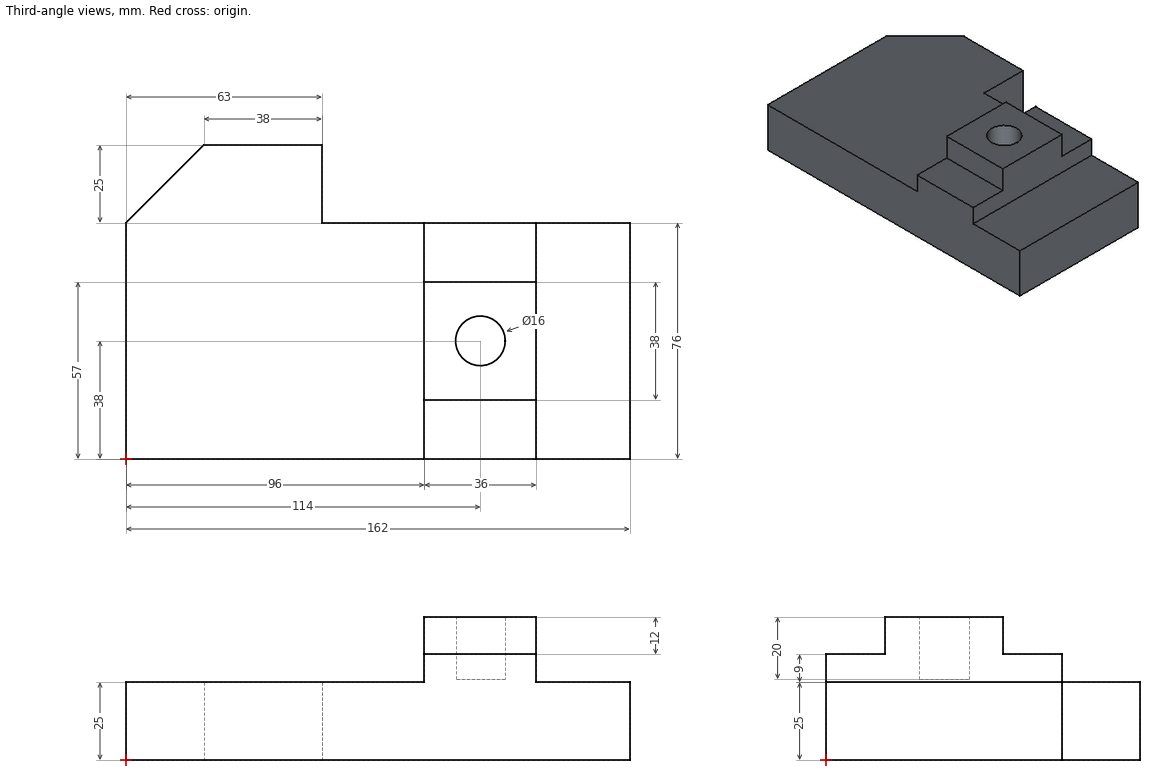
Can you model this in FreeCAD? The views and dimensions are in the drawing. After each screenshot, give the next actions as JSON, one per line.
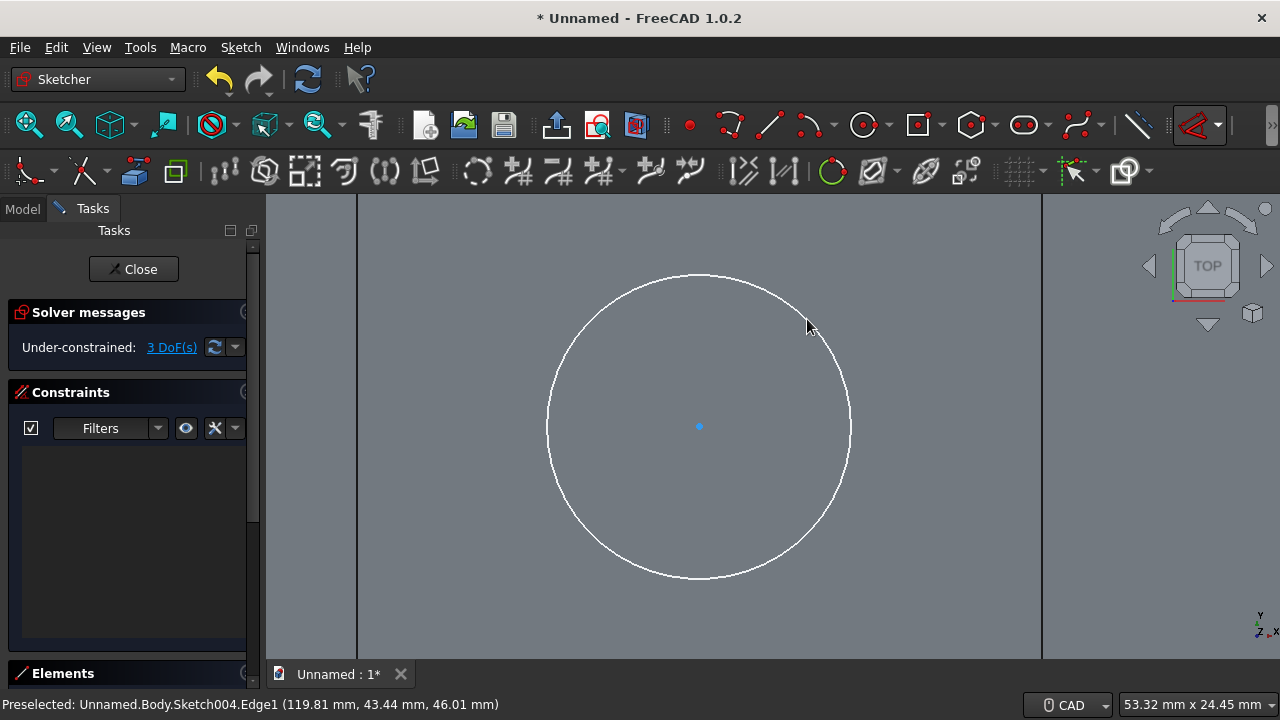
{"action": "left_click", "coordinate": [806, 319]}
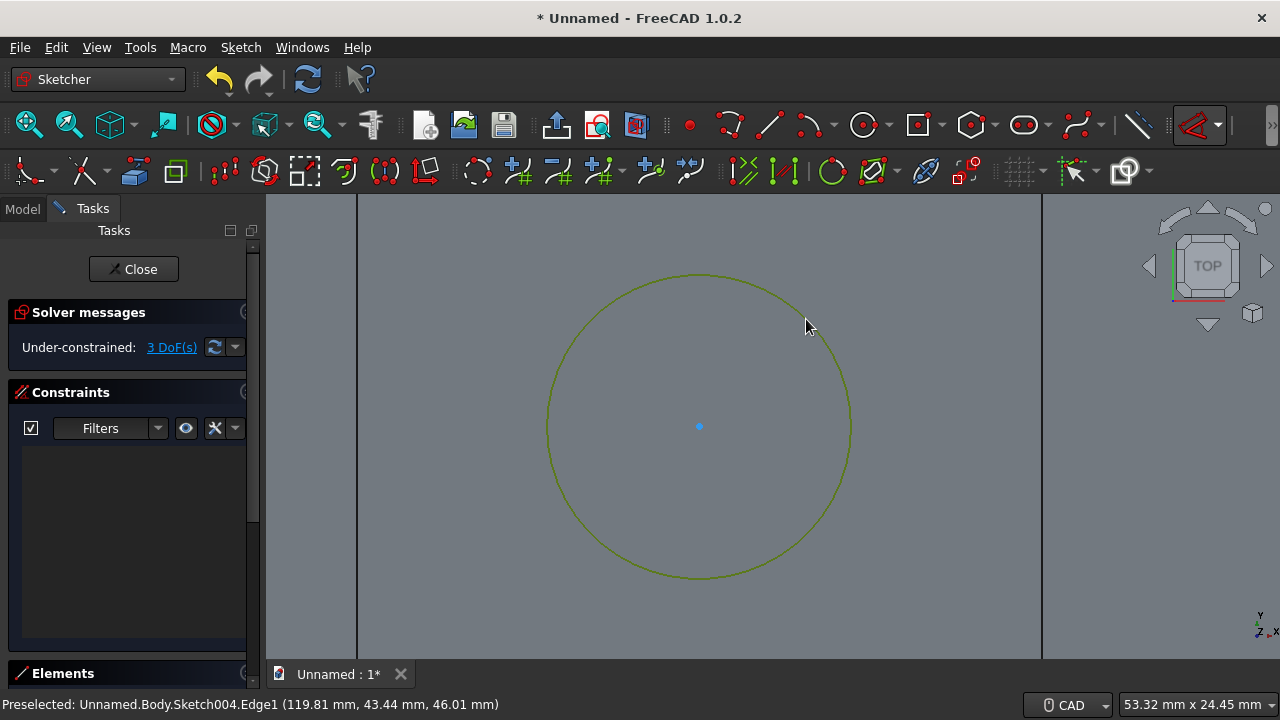
{"action": "key", "text": "k o"}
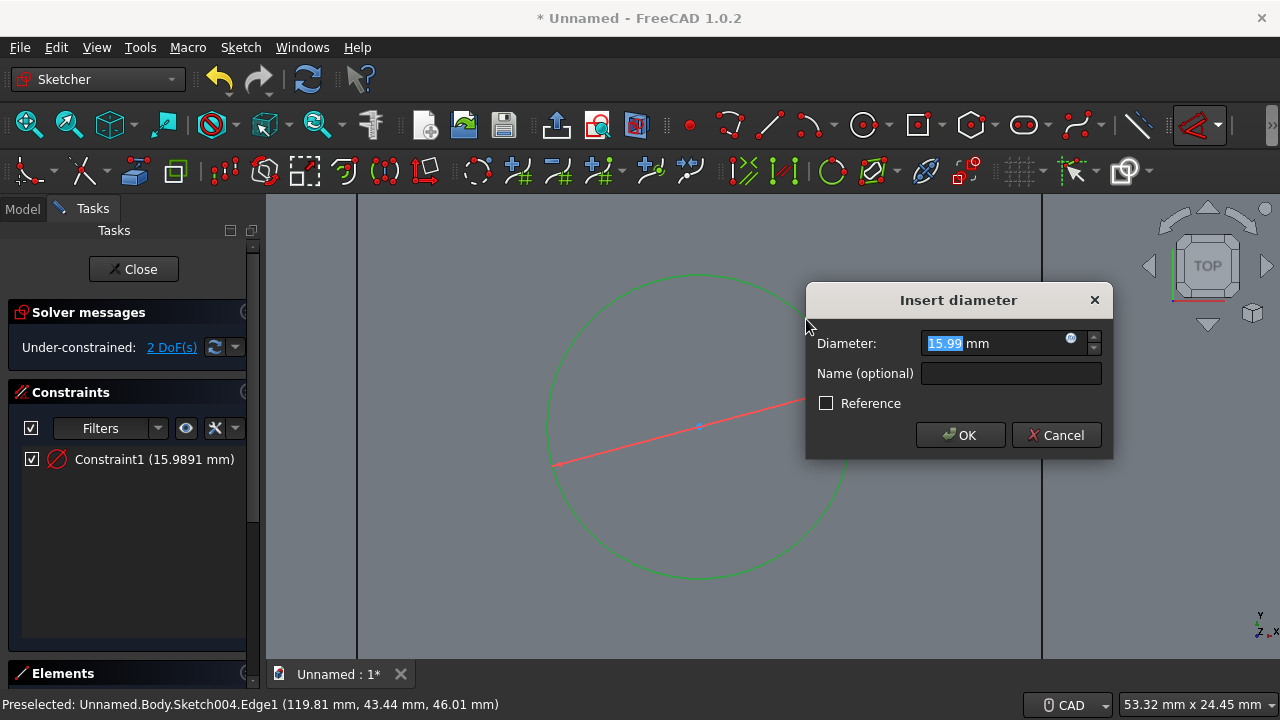
{"action": "type", "text": "16"}
{"action": "key", "text": "Return"}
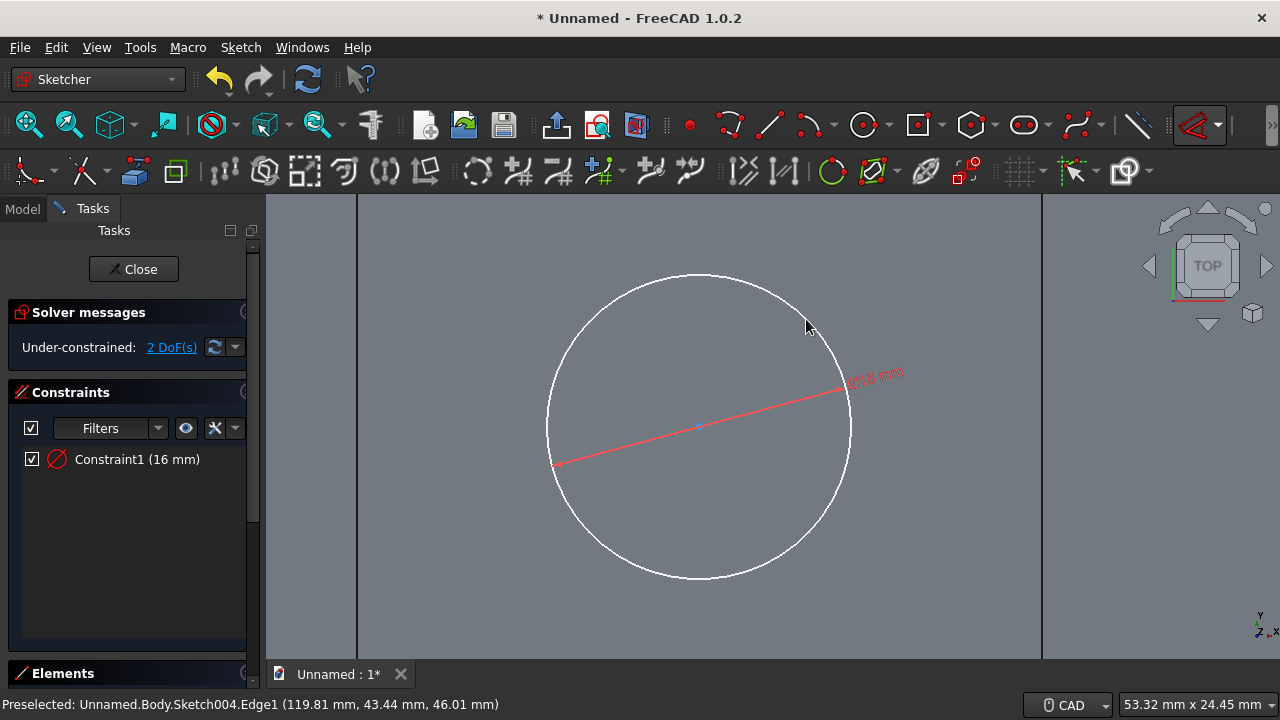
{"action": "left_click", "coordinate": [699, 427]}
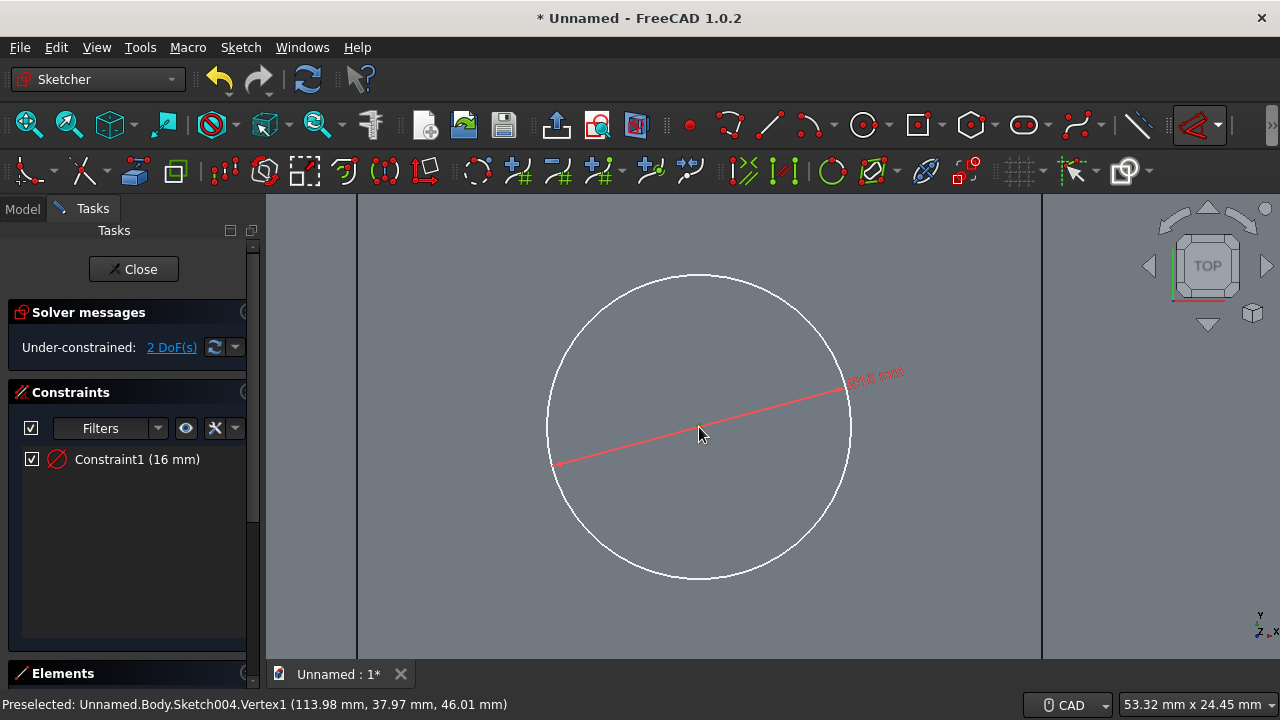
{"action": "key", "text": "i"}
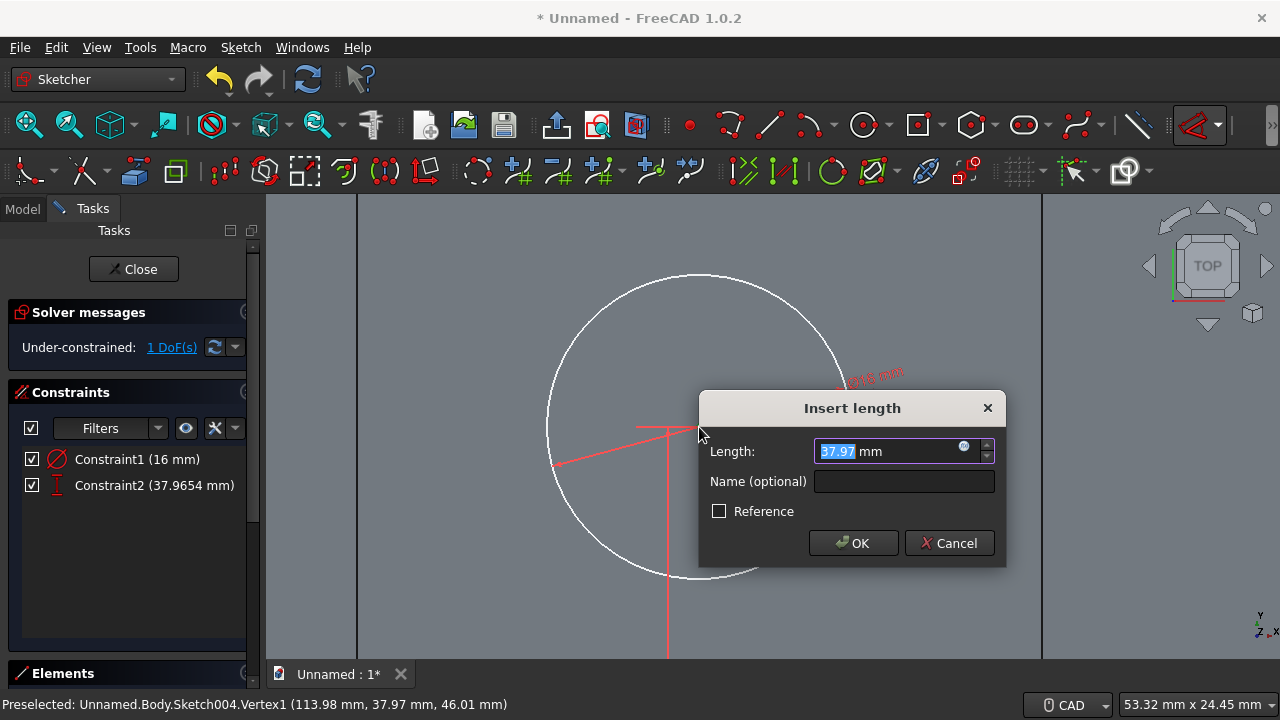
{"action": "type", "text": "38"}
{"action": "key", "text": "Return"}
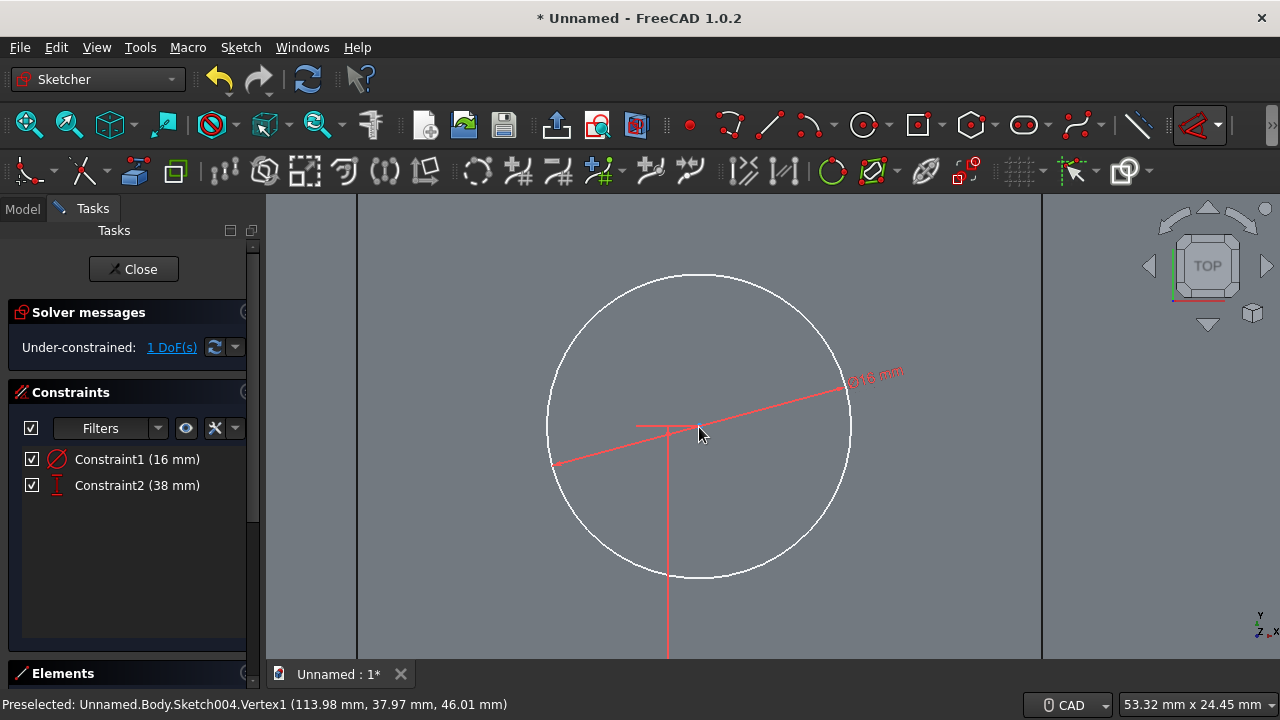
{"action": "left_click", "coordinate": [699, 426]}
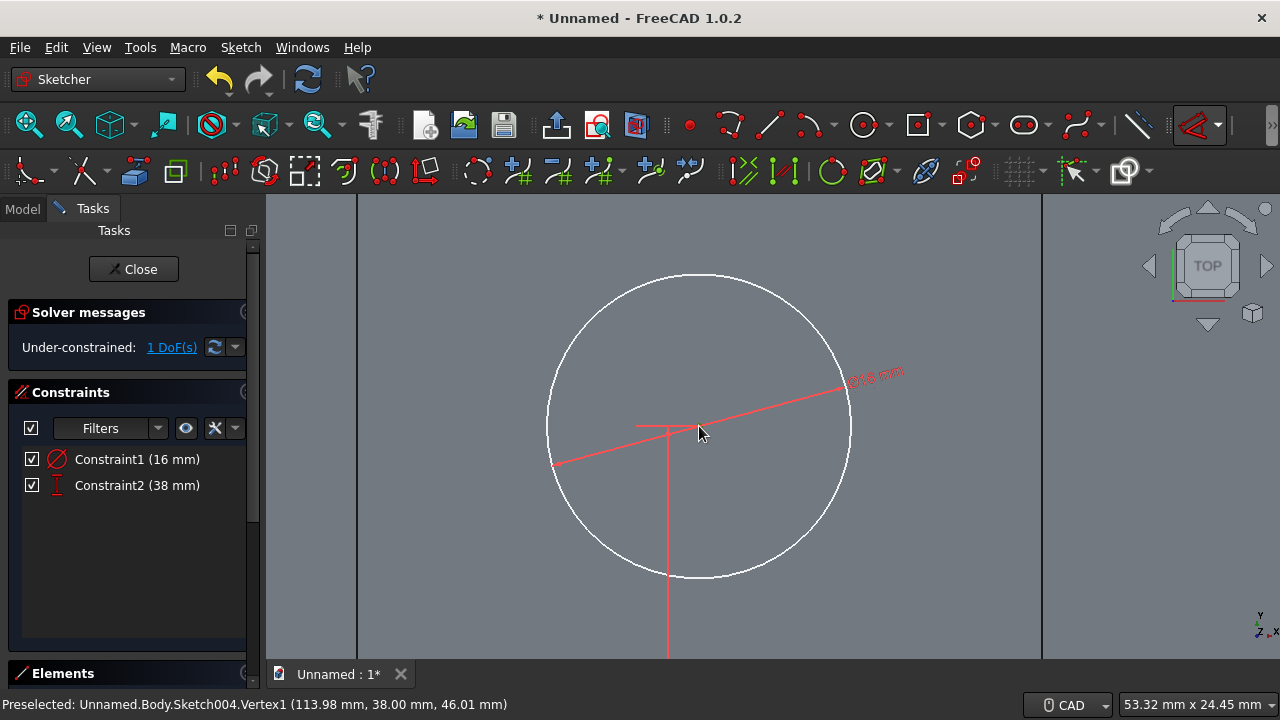
{"action": "key", "text": "l"}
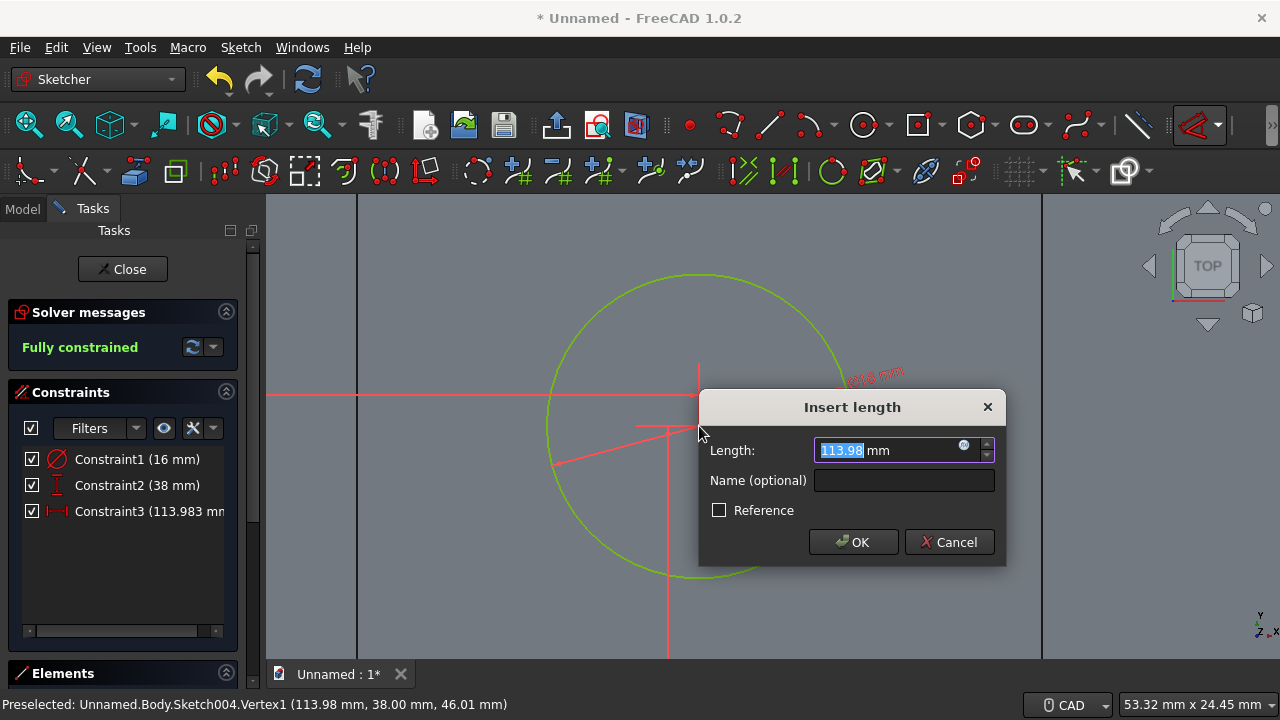
{"action": "type", "text": "114"}
{"action": "key", "text": "Return"}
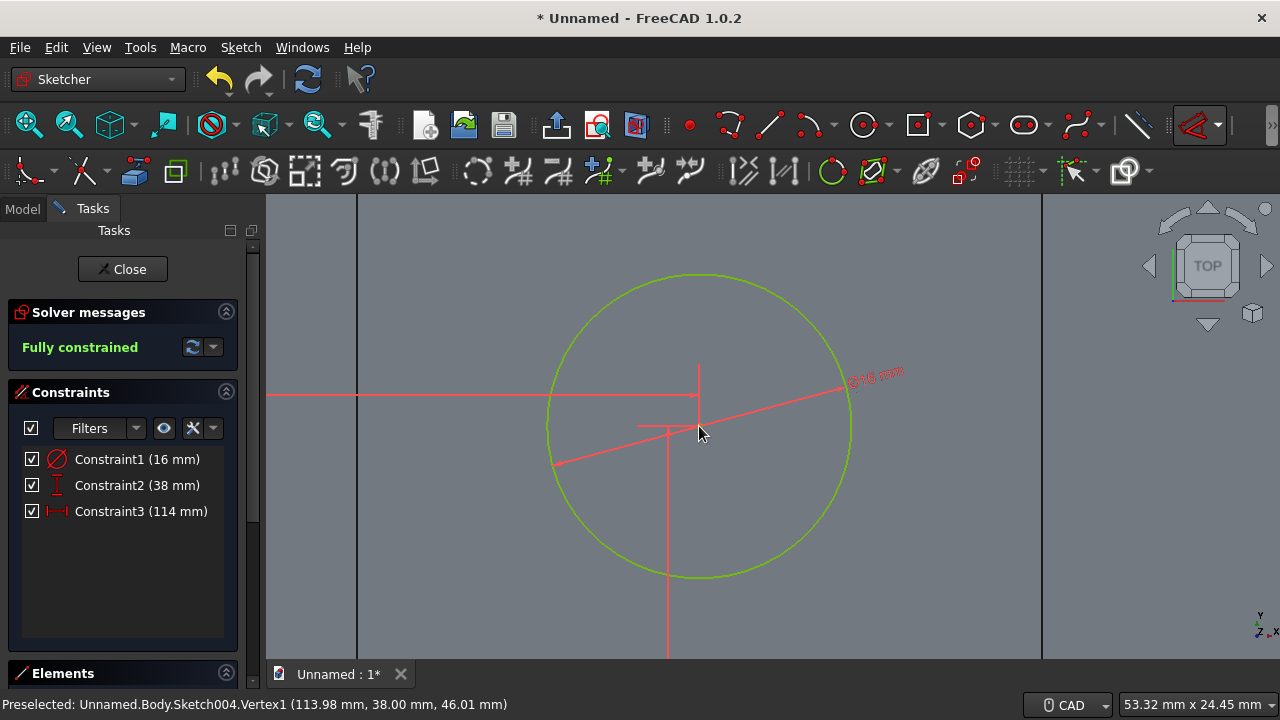
{"action": "left_click", "coordinate": [123, 269]}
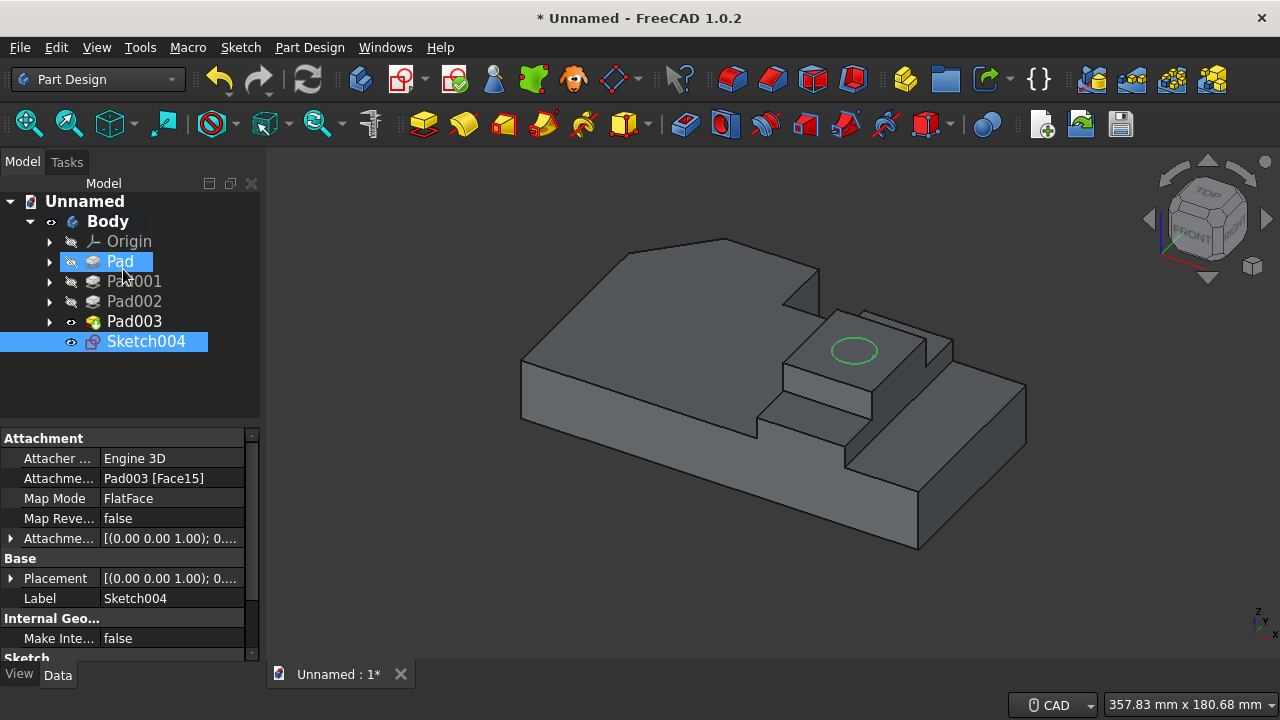
{"action": "left_click", "coordinate": [686, 124]}